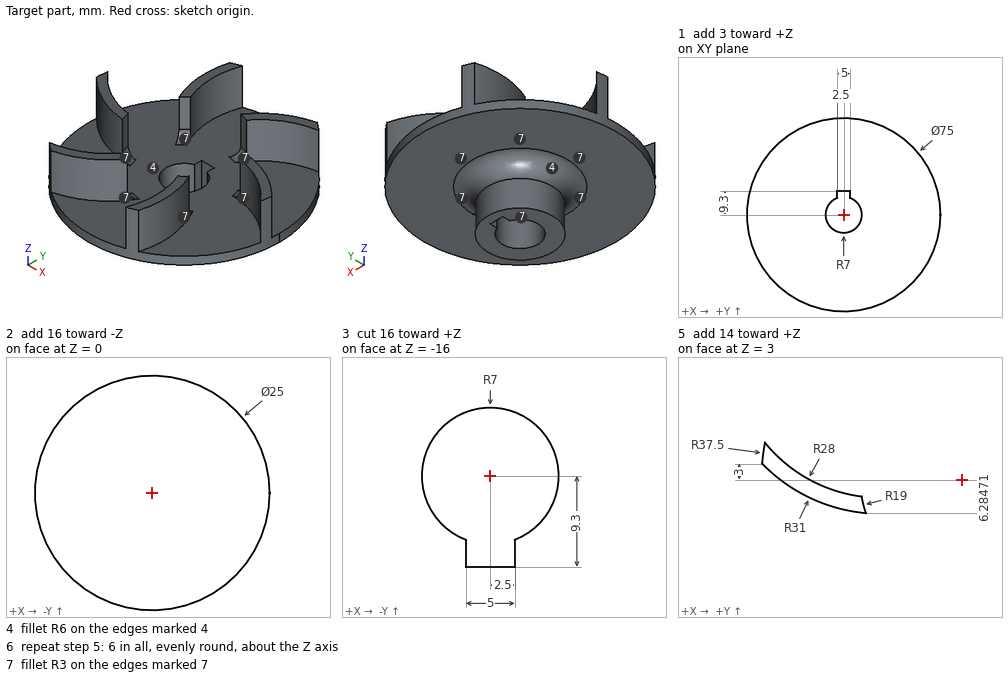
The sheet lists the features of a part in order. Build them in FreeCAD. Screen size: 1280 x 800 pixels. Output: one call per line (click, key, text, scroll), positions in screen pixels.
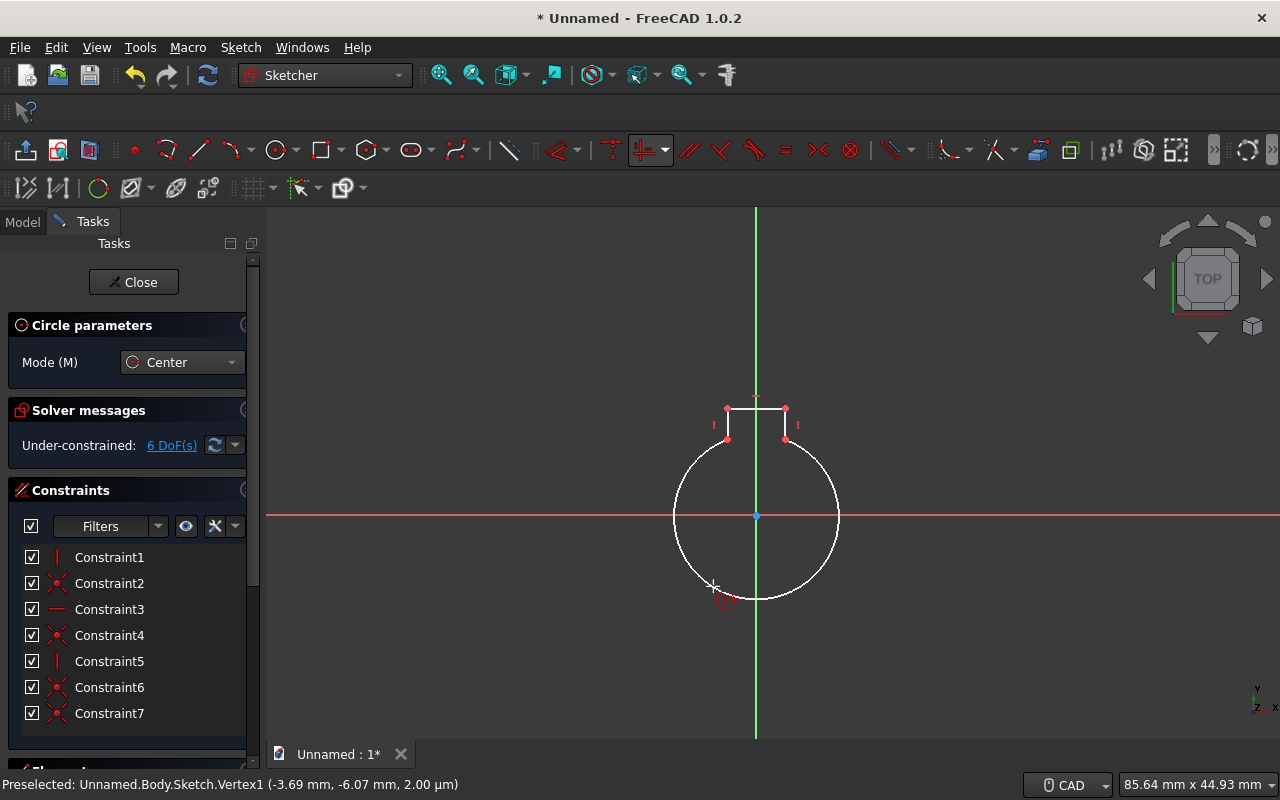
click(756, 515)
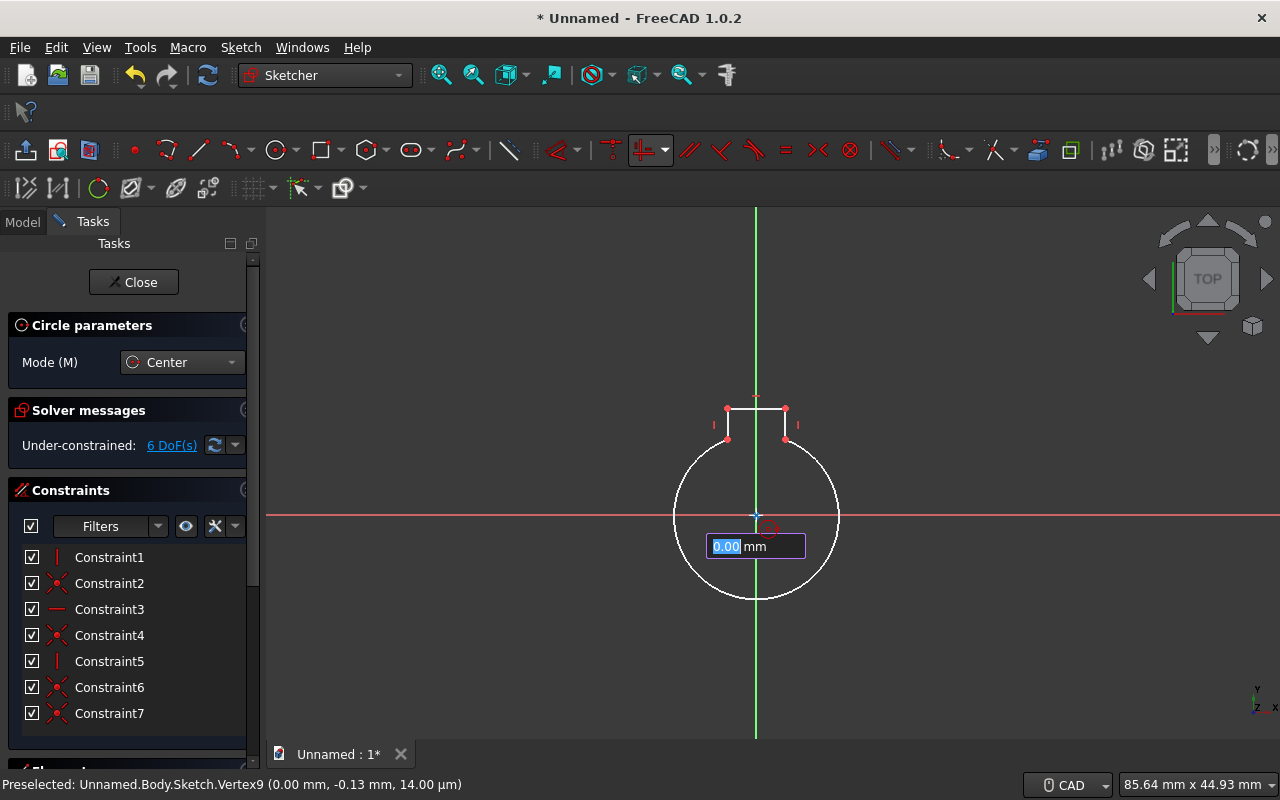
scroll(674, 448, down, 5)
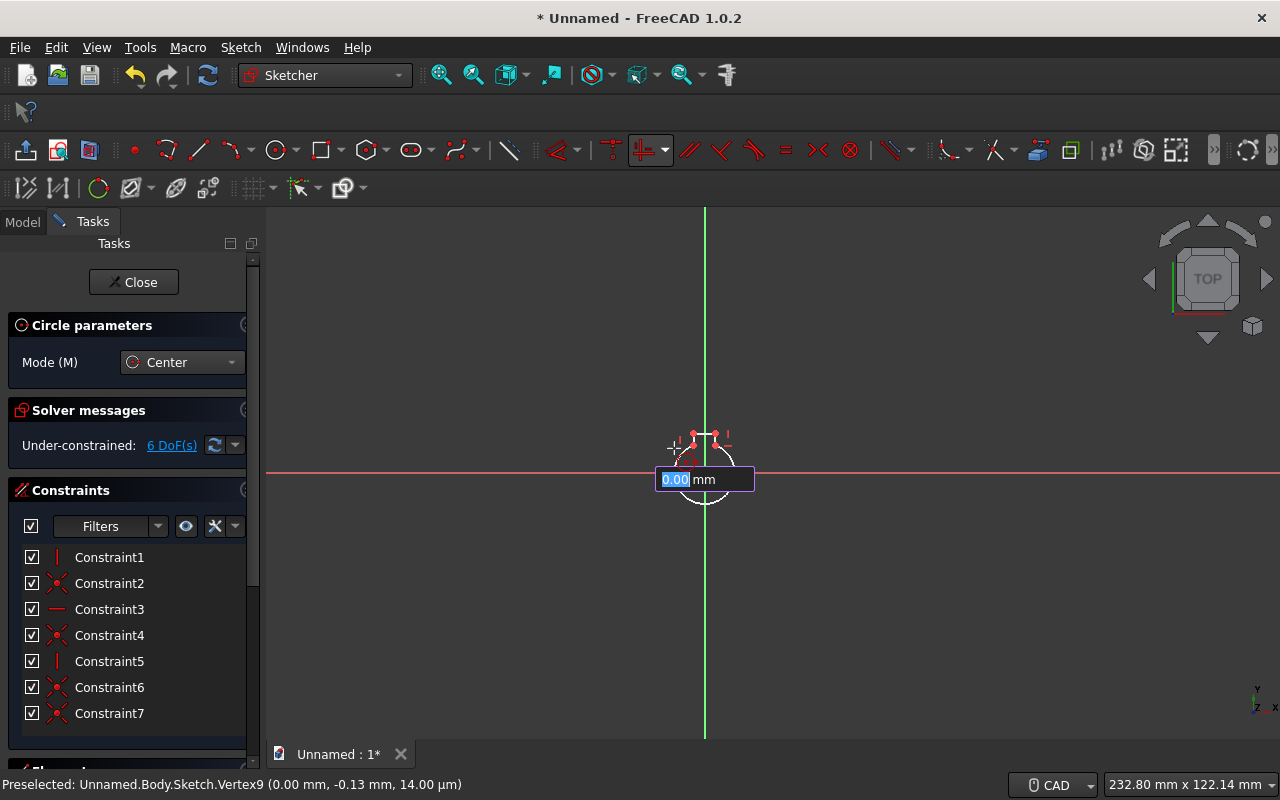
click(820, 358)
key(Escape)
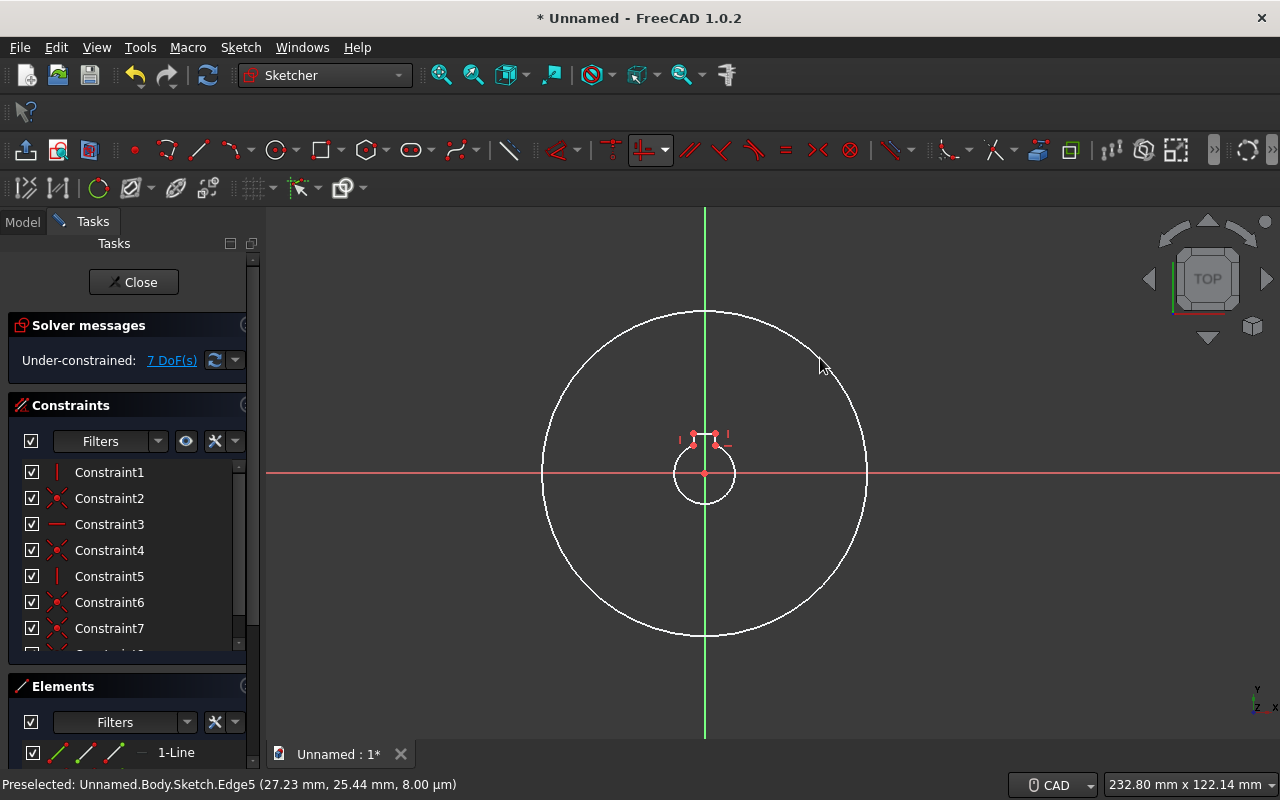
scroll(705, 473, up, 2)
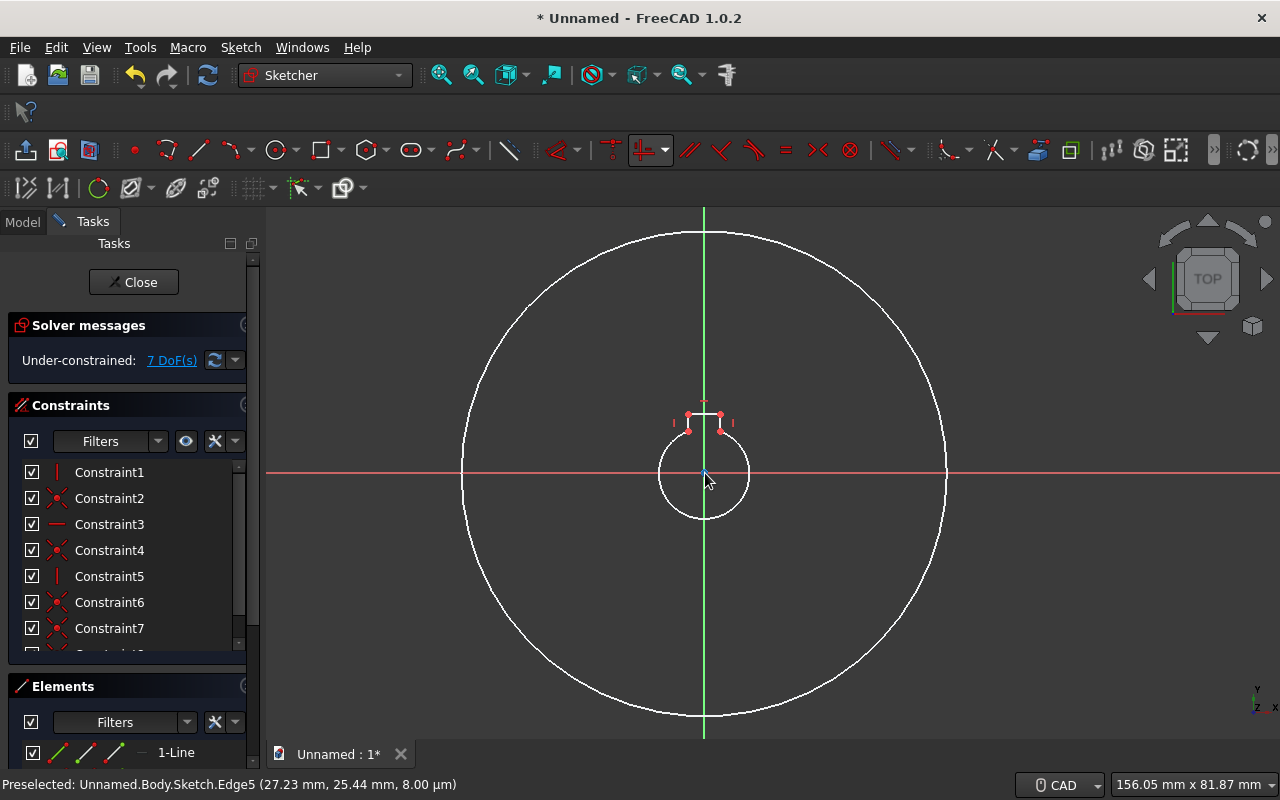
drag(694, 463, 714, 484)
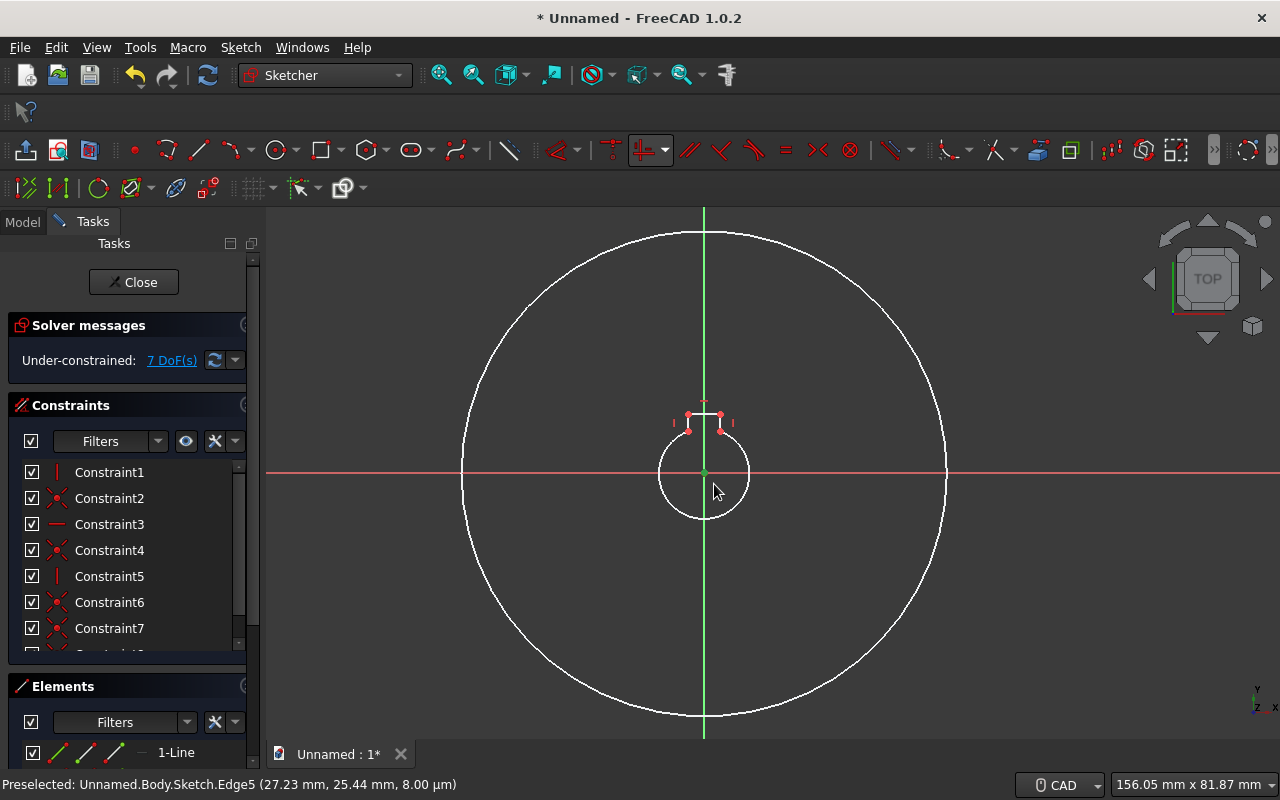
key(c)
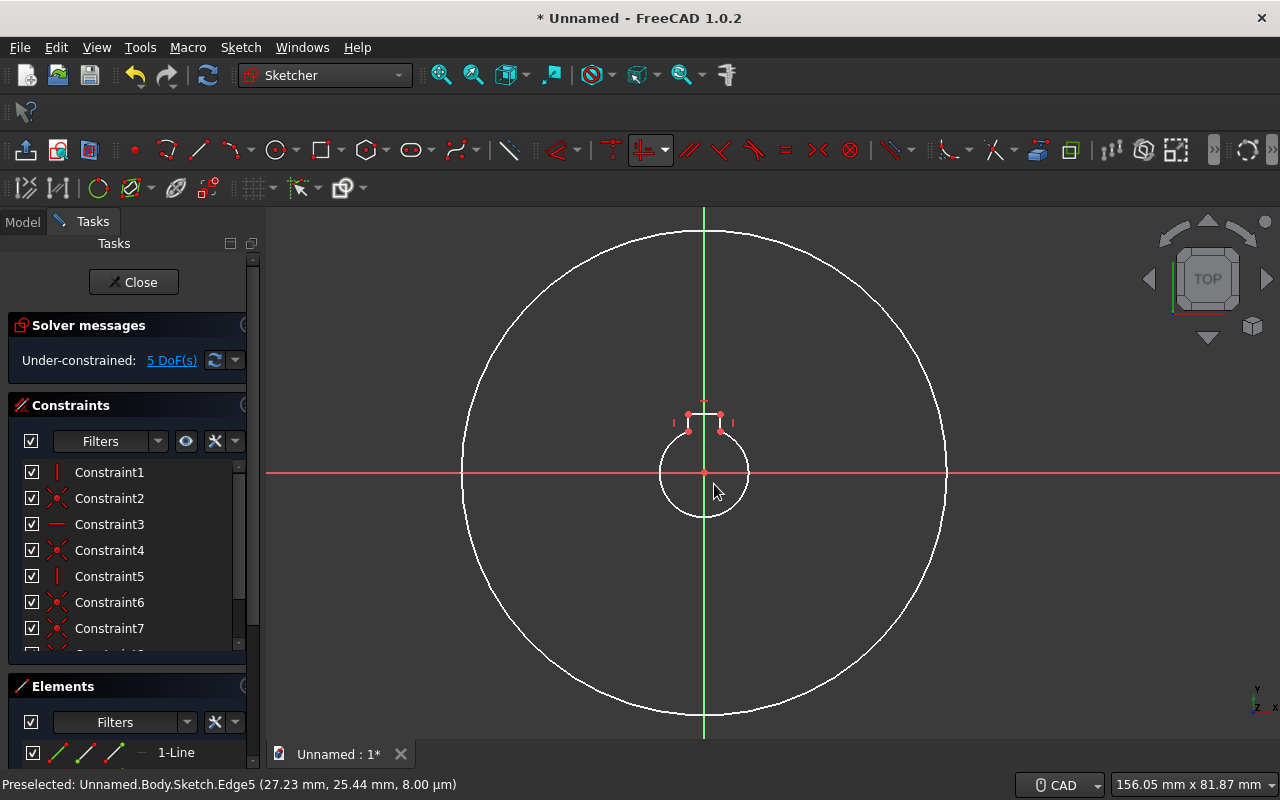
click(664, 493)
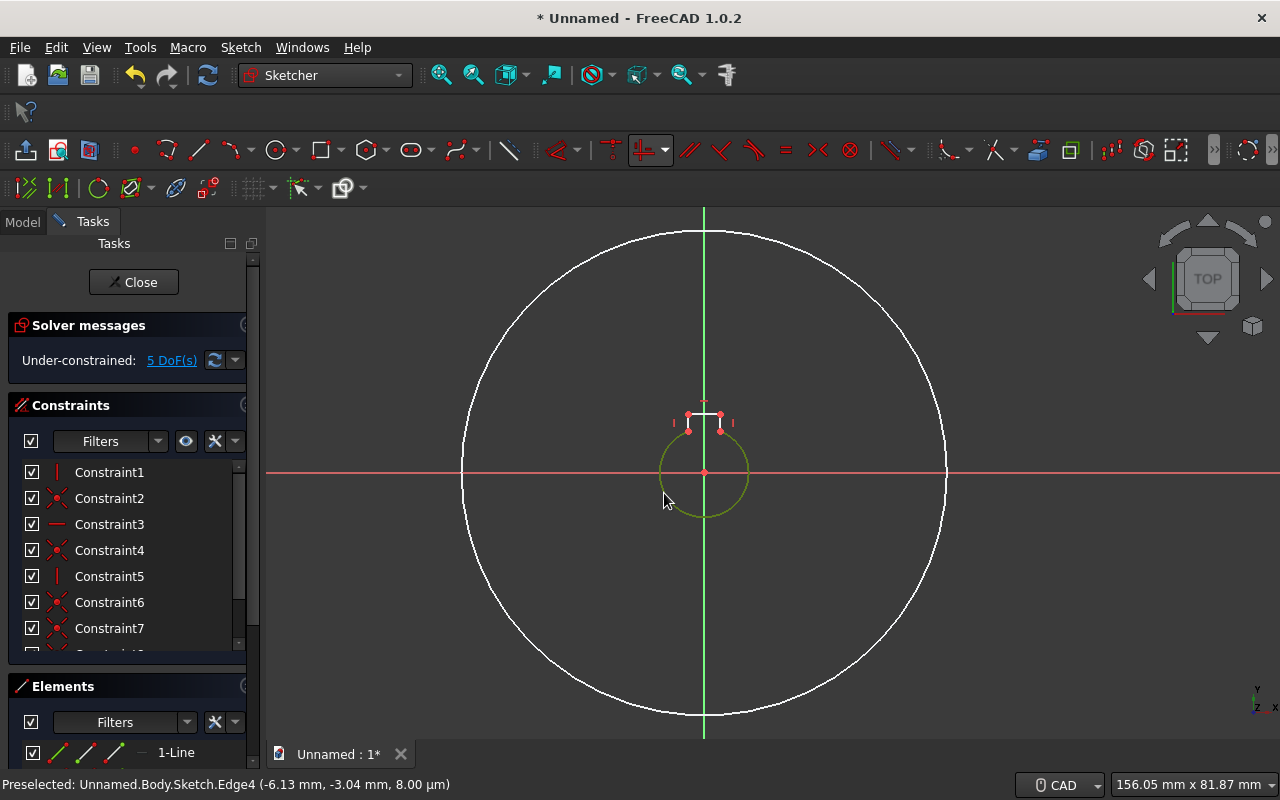
key(k)
key(r)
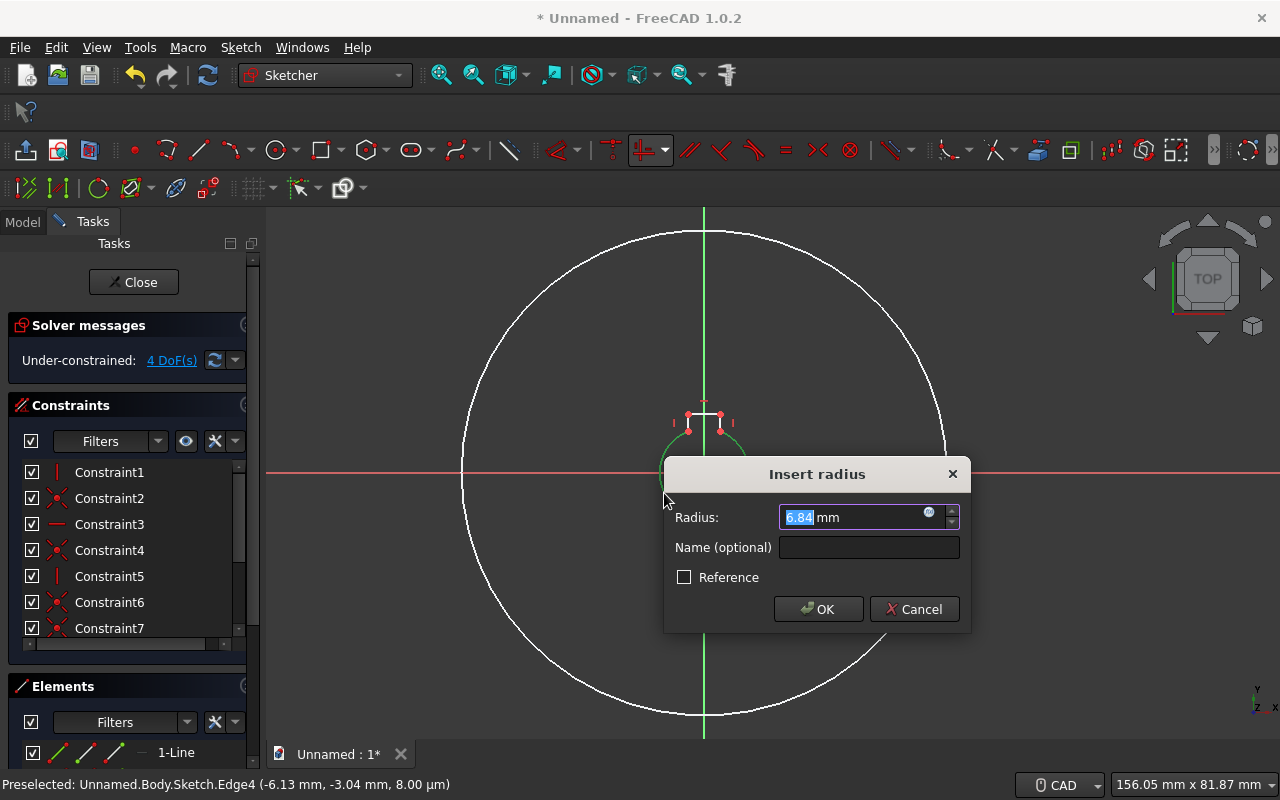
text(7)
key(Return)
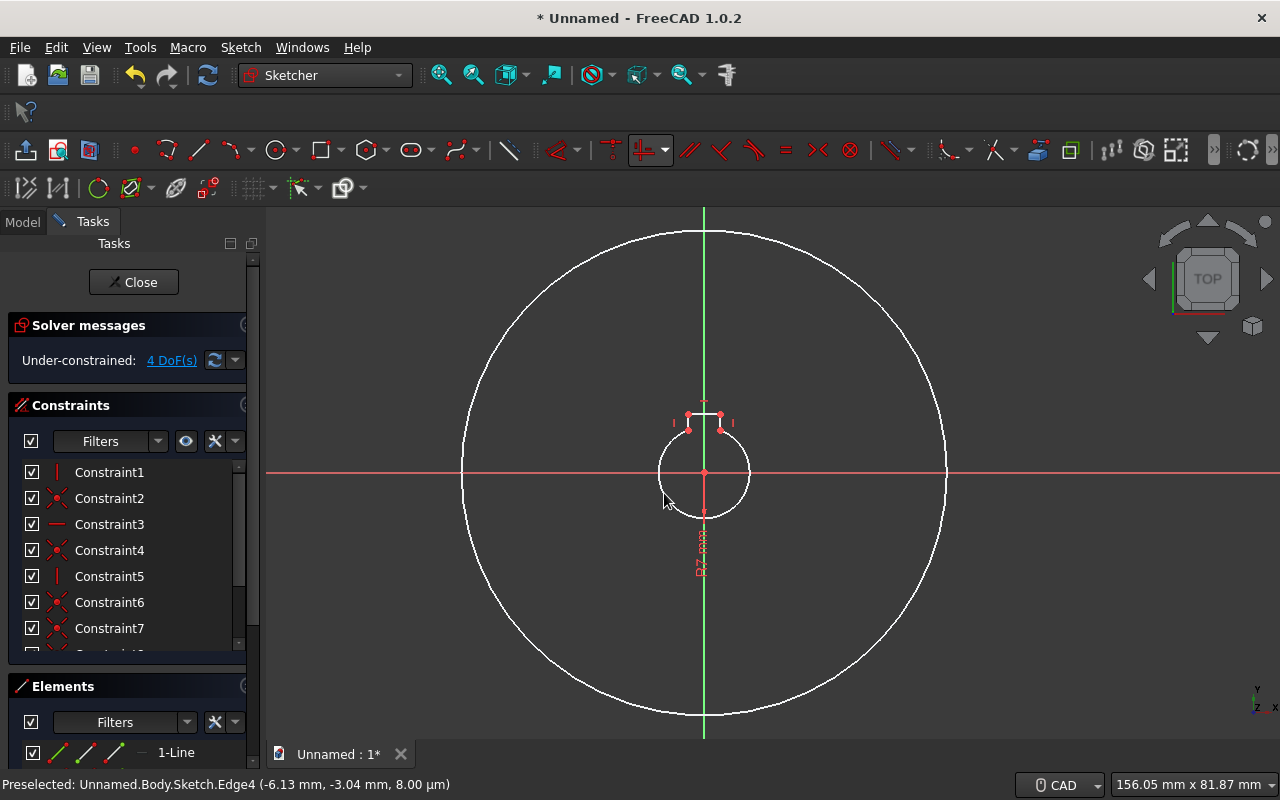
click(875, 301)